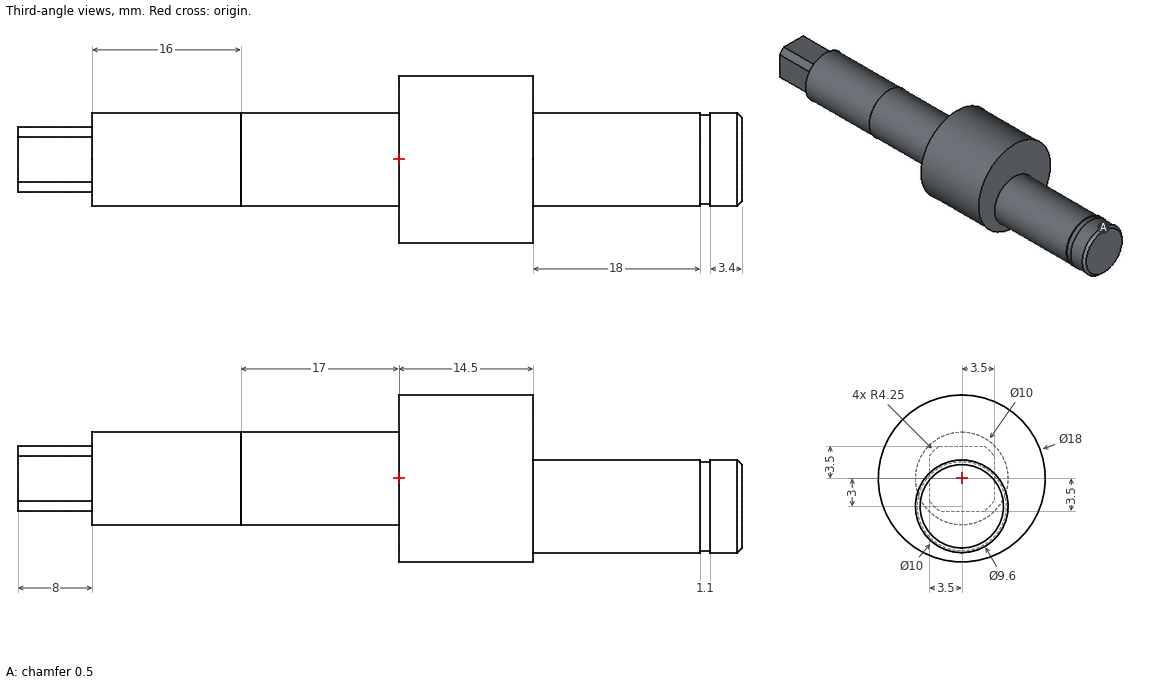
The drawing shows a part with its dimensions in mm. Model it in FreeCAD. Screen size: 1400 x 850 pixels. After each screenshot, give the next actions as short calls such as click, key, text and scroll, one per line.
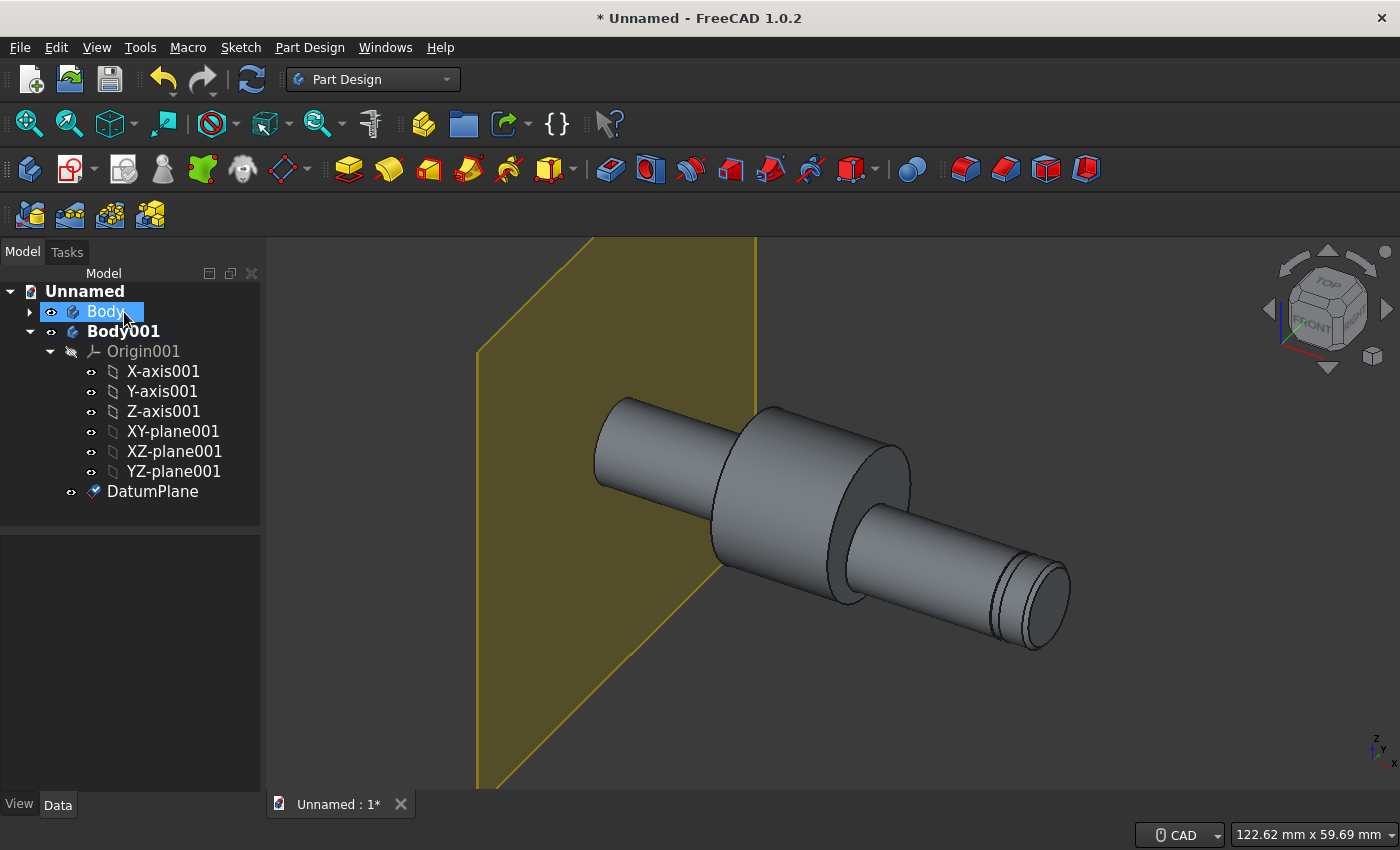
click(116, 492)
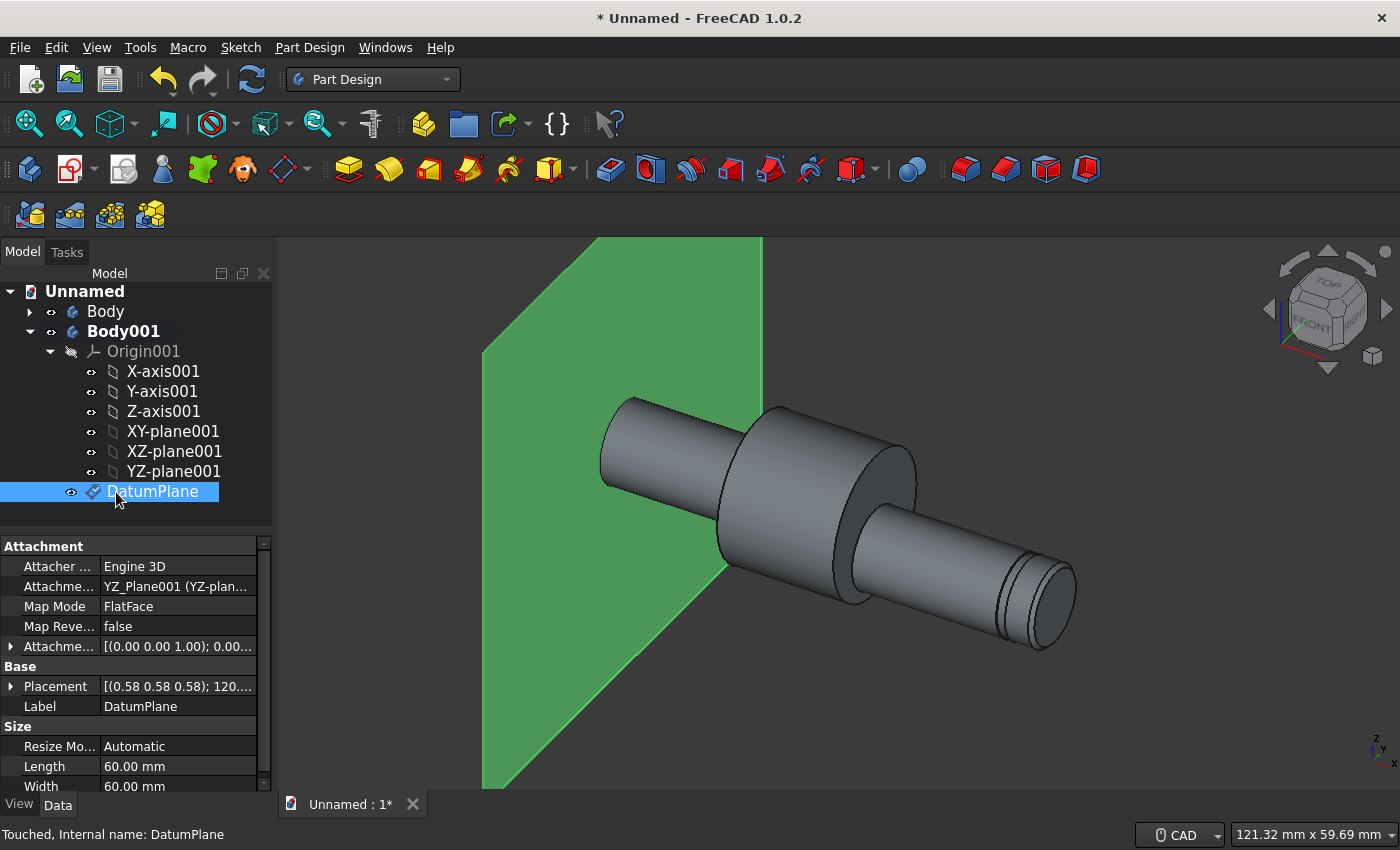
click(70, 170)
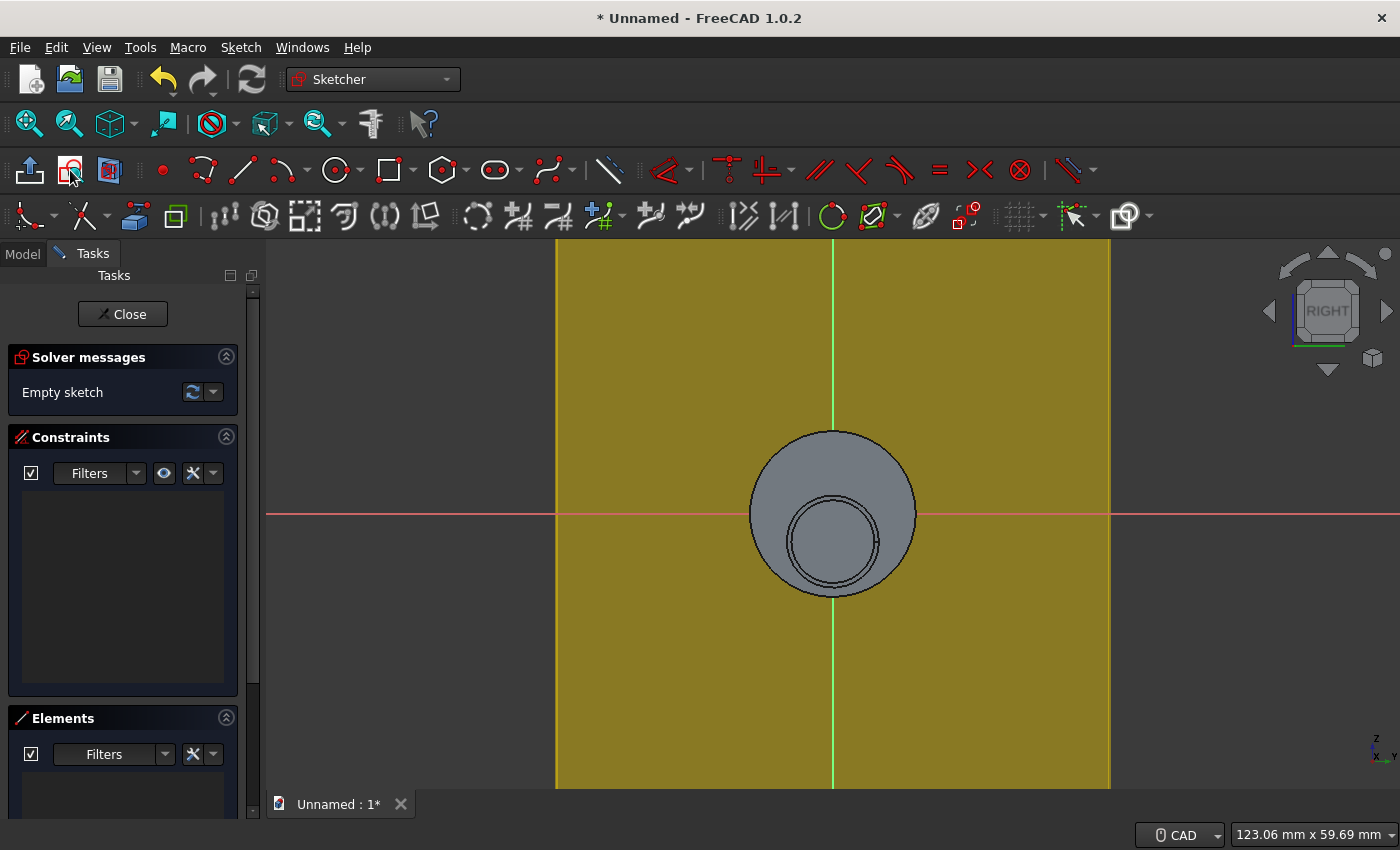
scroll(855, 514, up, 7)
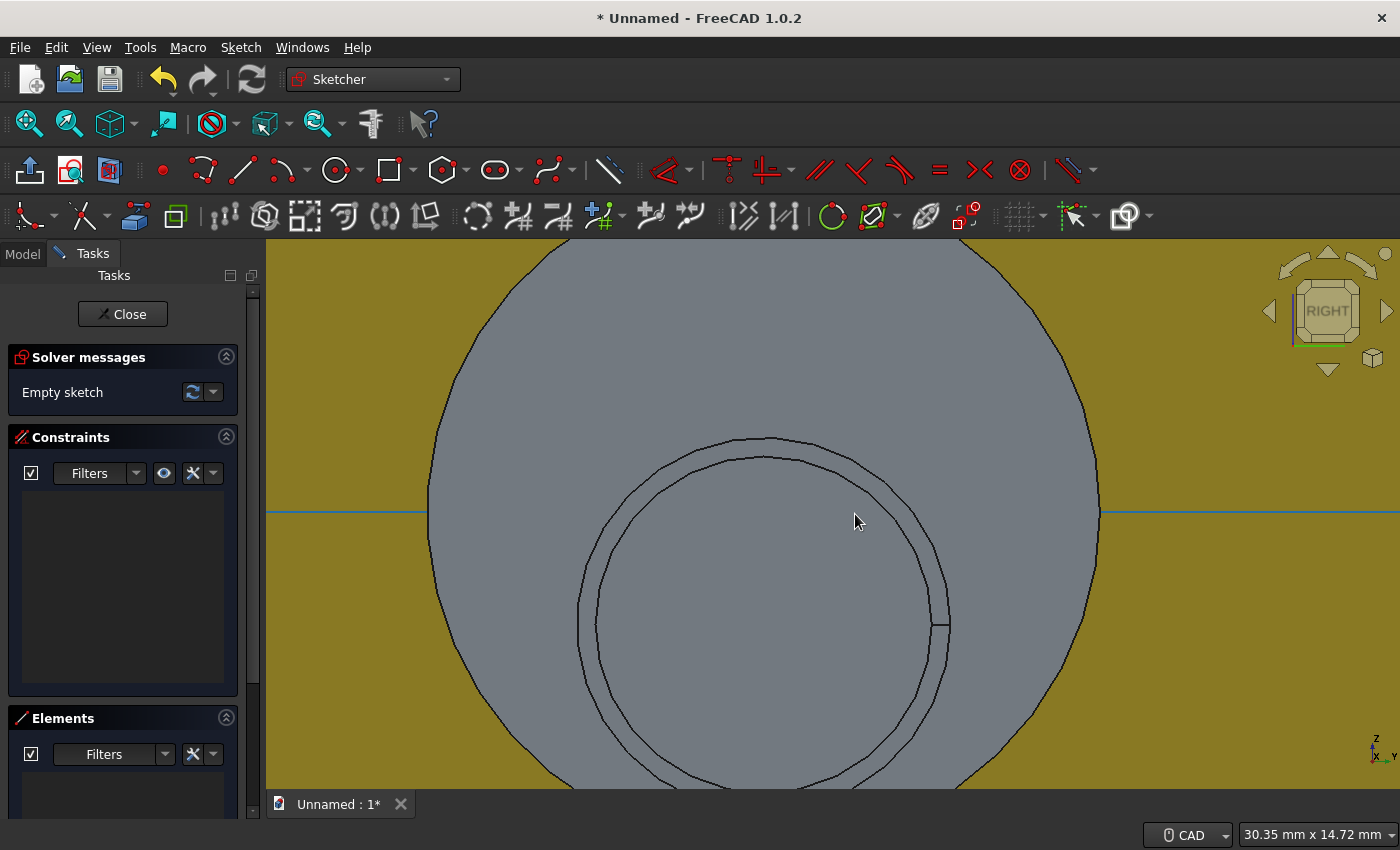
click(336, 170)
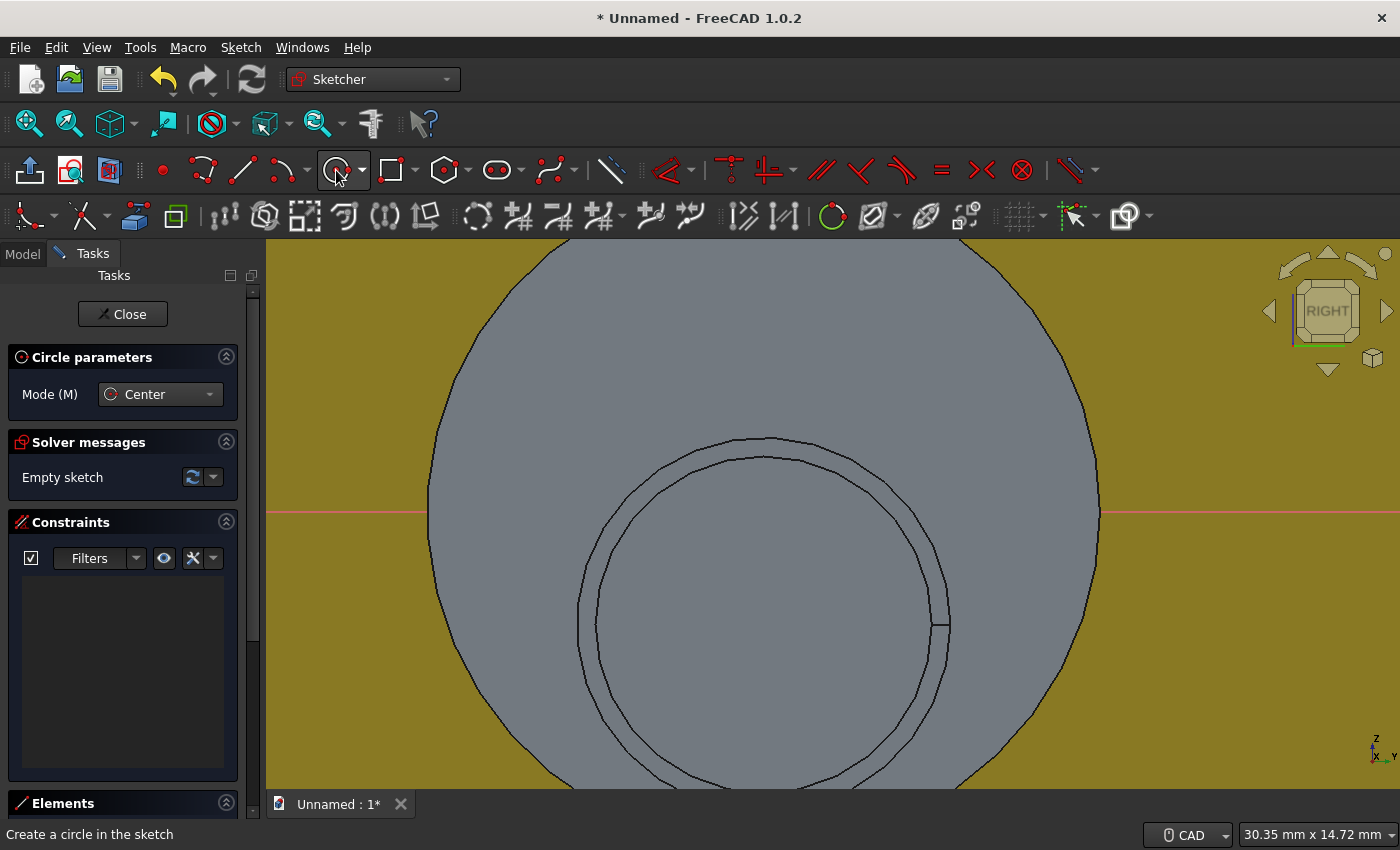
click(764, 512)
move(896, 380)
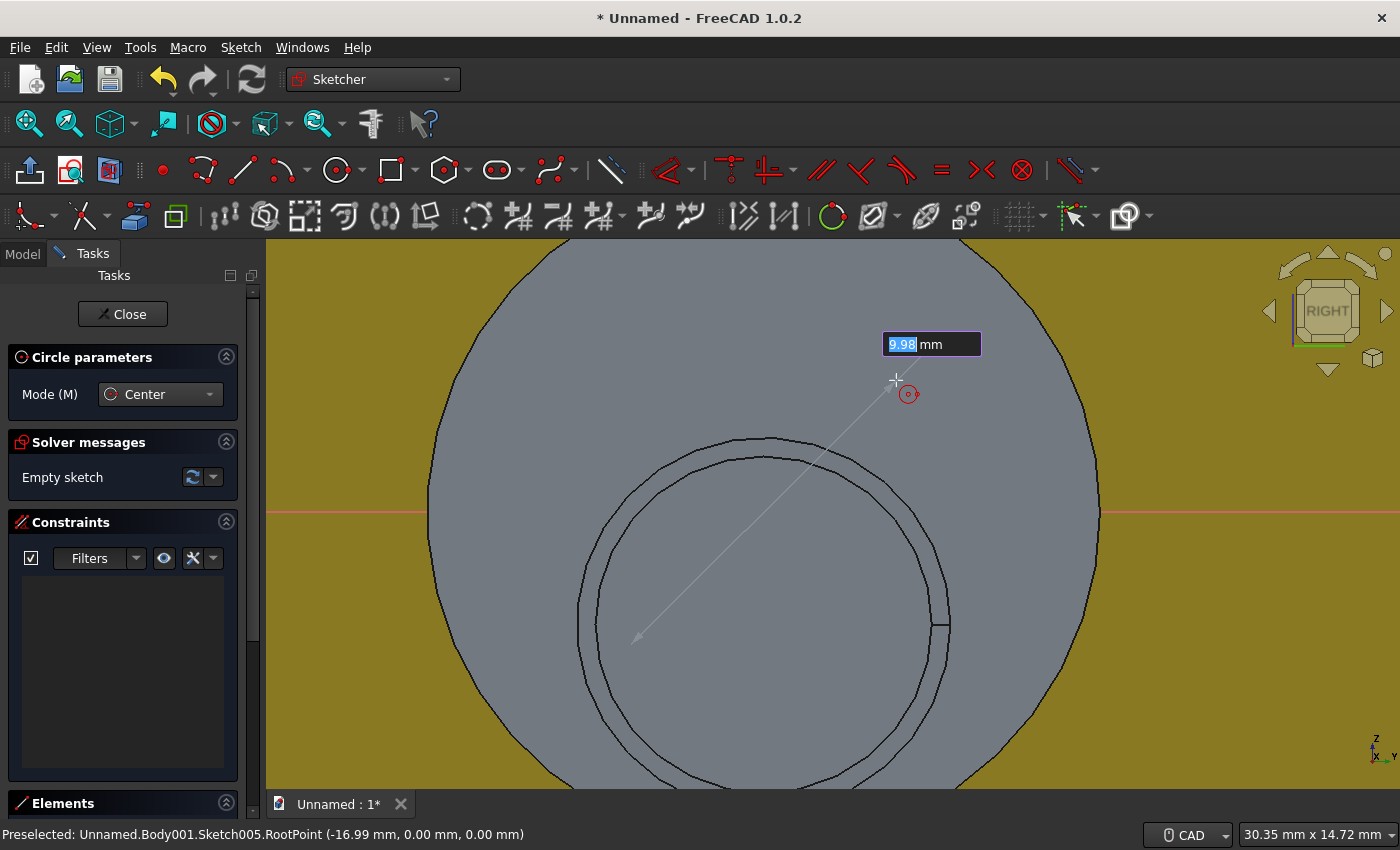
text(10)
key(Return)
key(Escape)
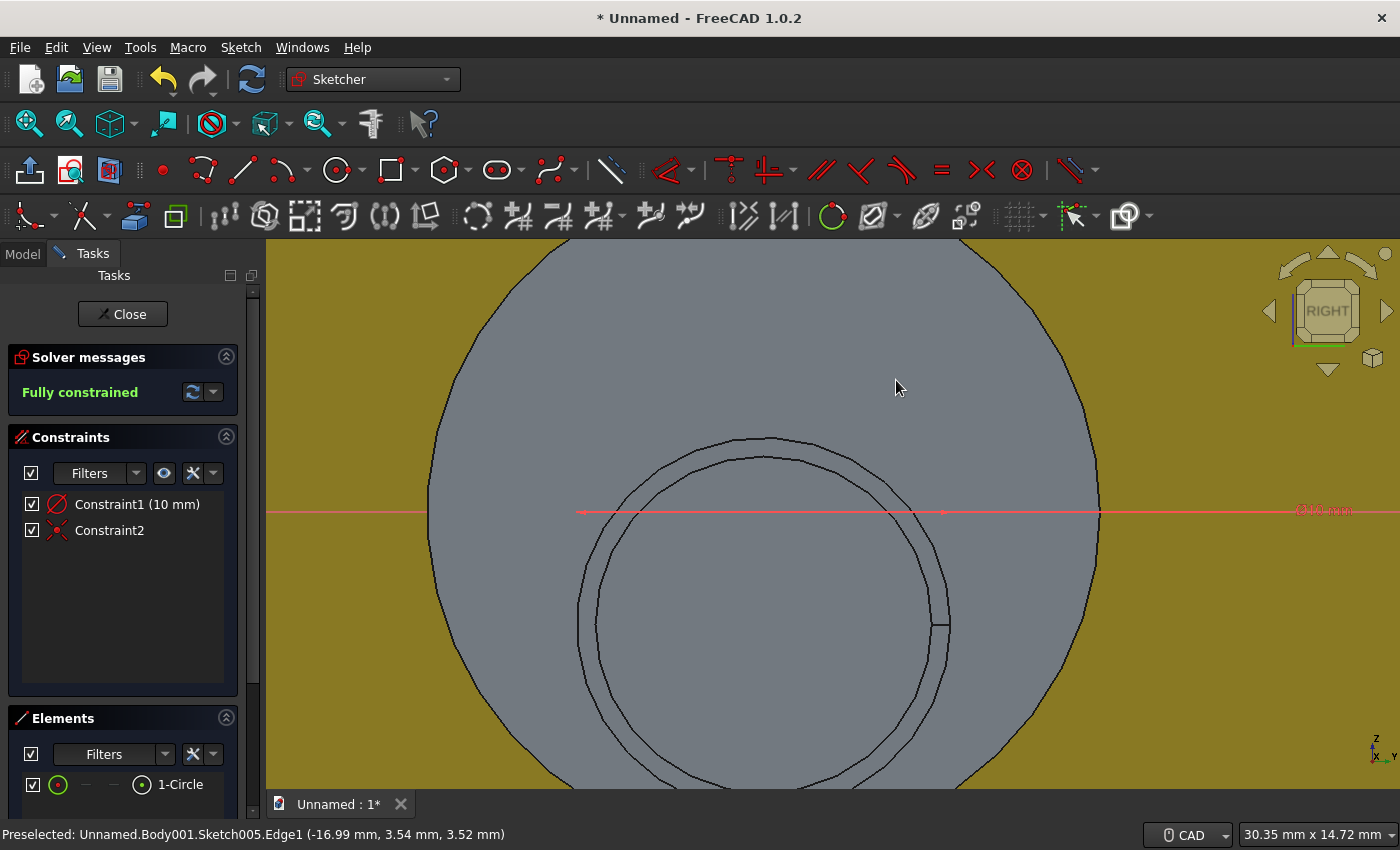
click(123, 314)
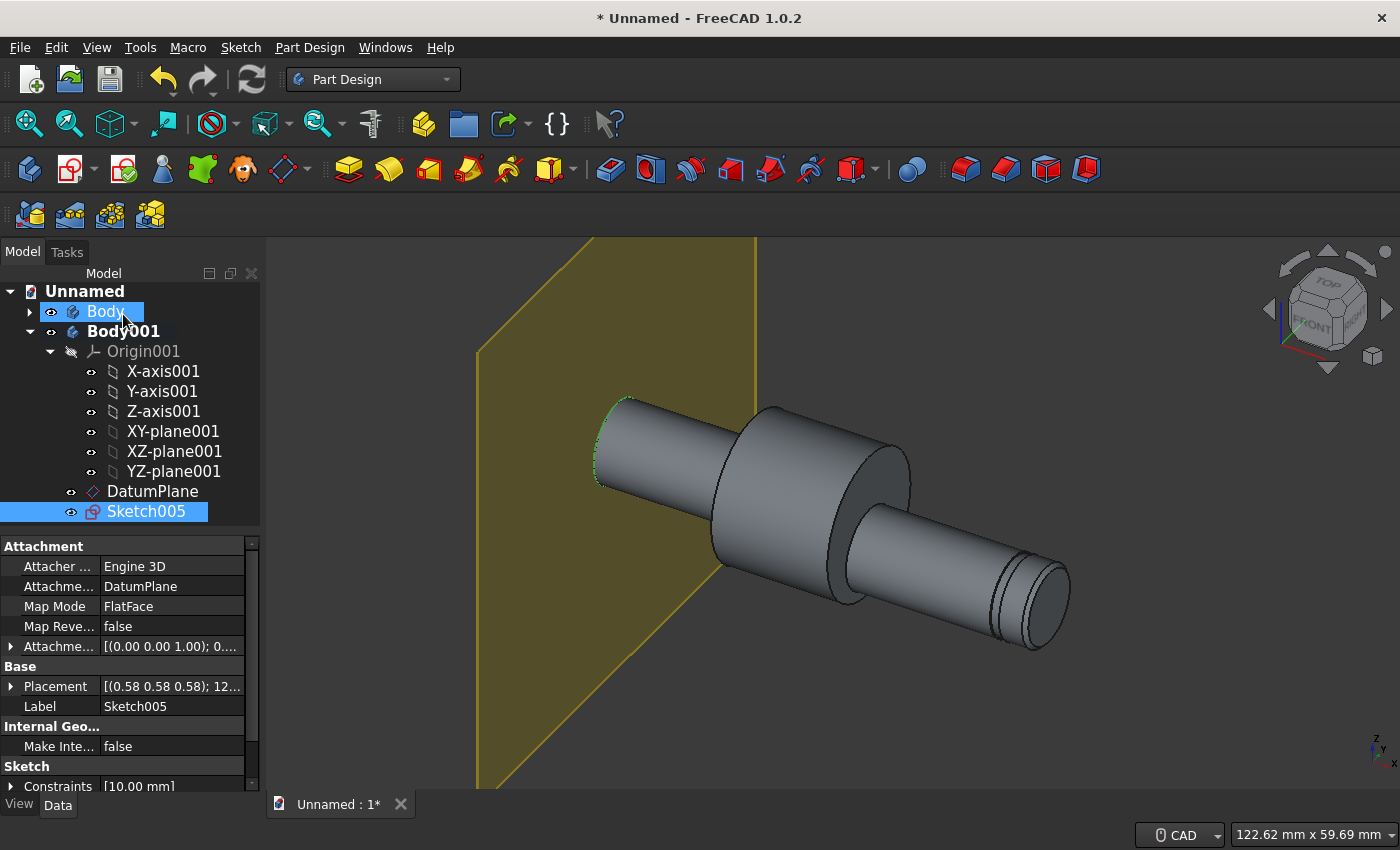
click(350, 170)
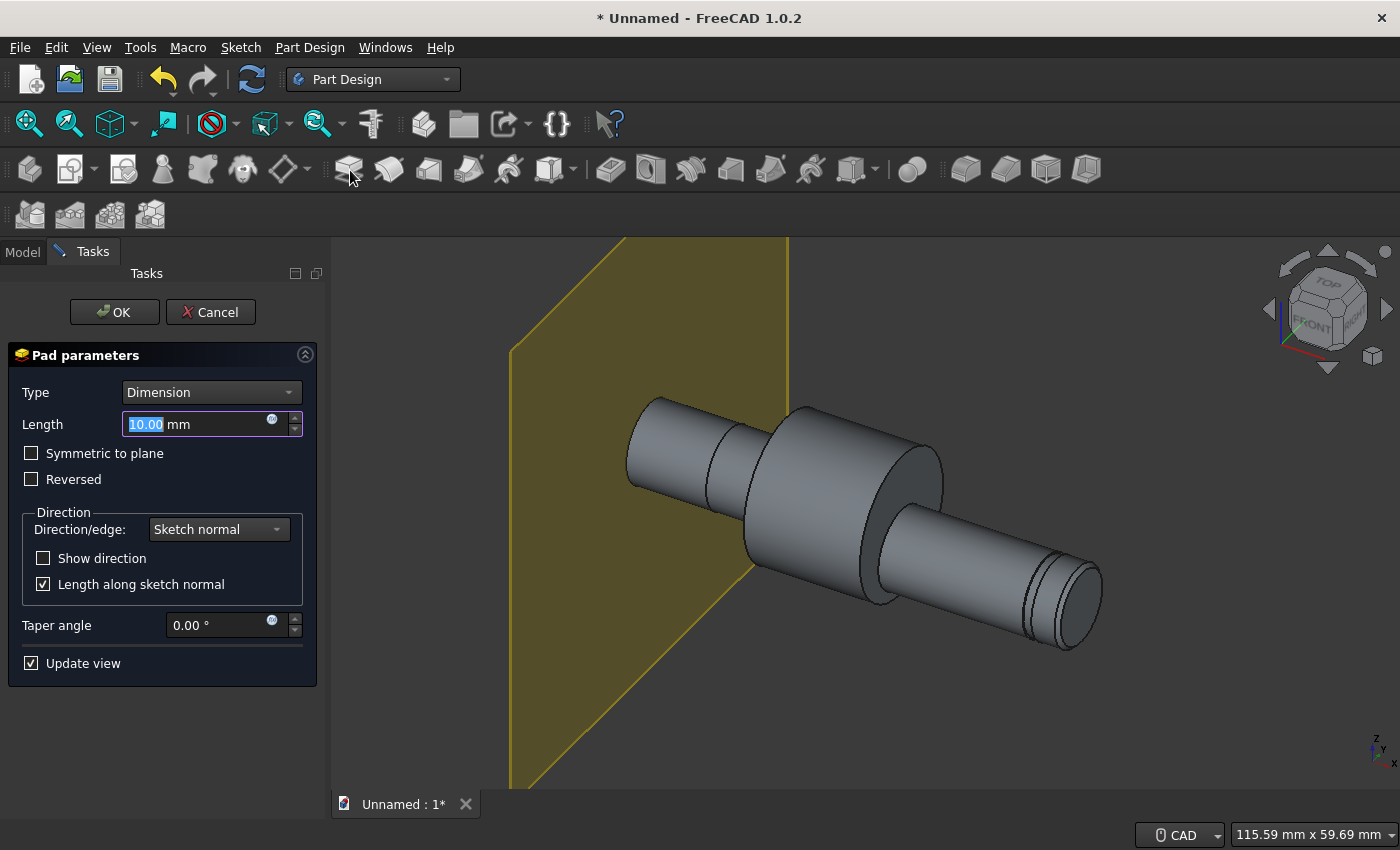
text(16)
key(Tab)